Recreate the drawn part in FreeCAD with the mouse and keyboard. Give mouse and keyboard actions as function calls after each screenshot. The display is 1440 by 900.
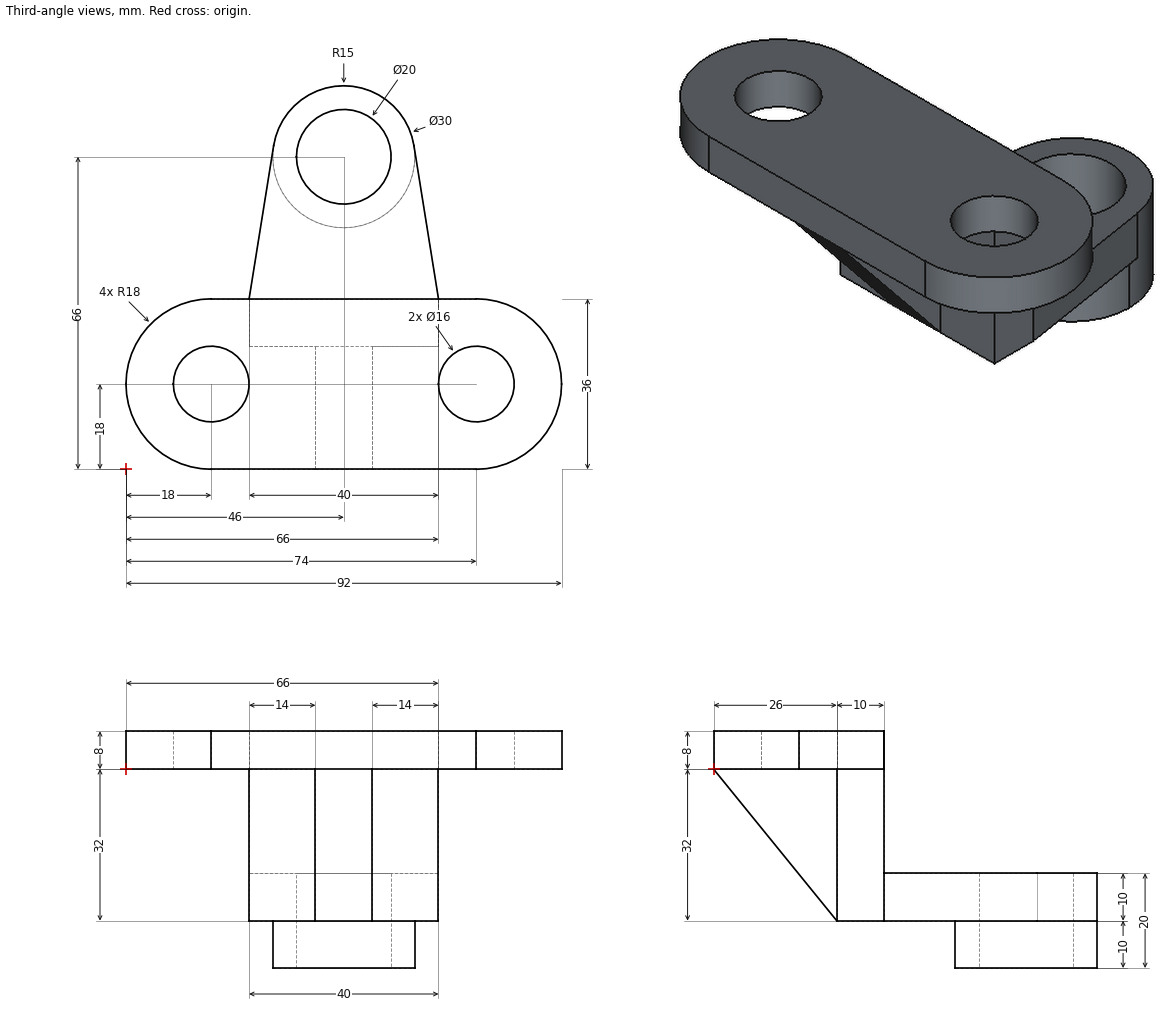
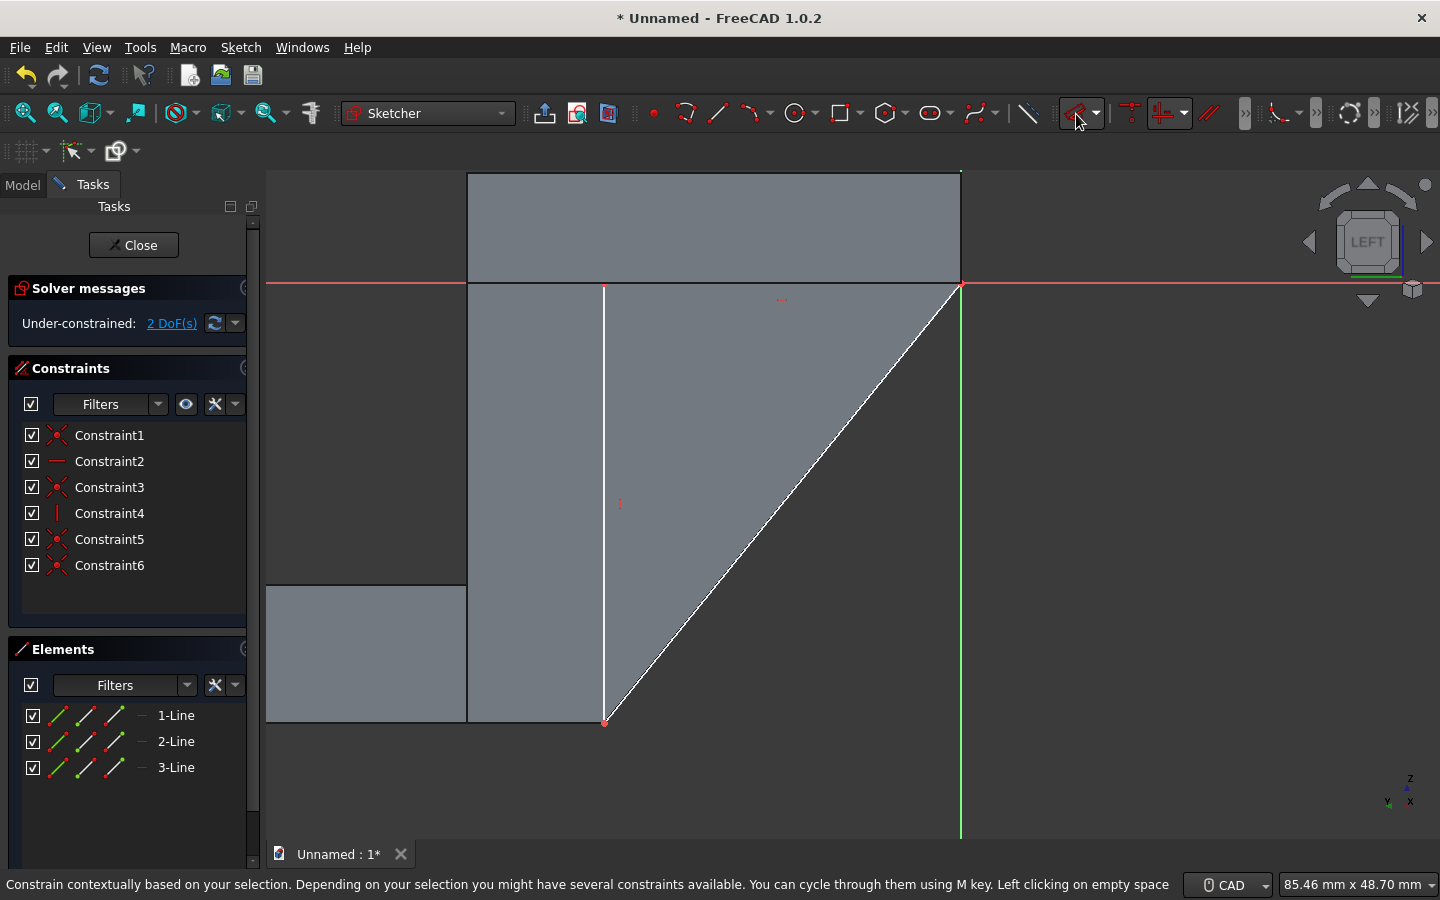
click(854, 283)
click(783, 249)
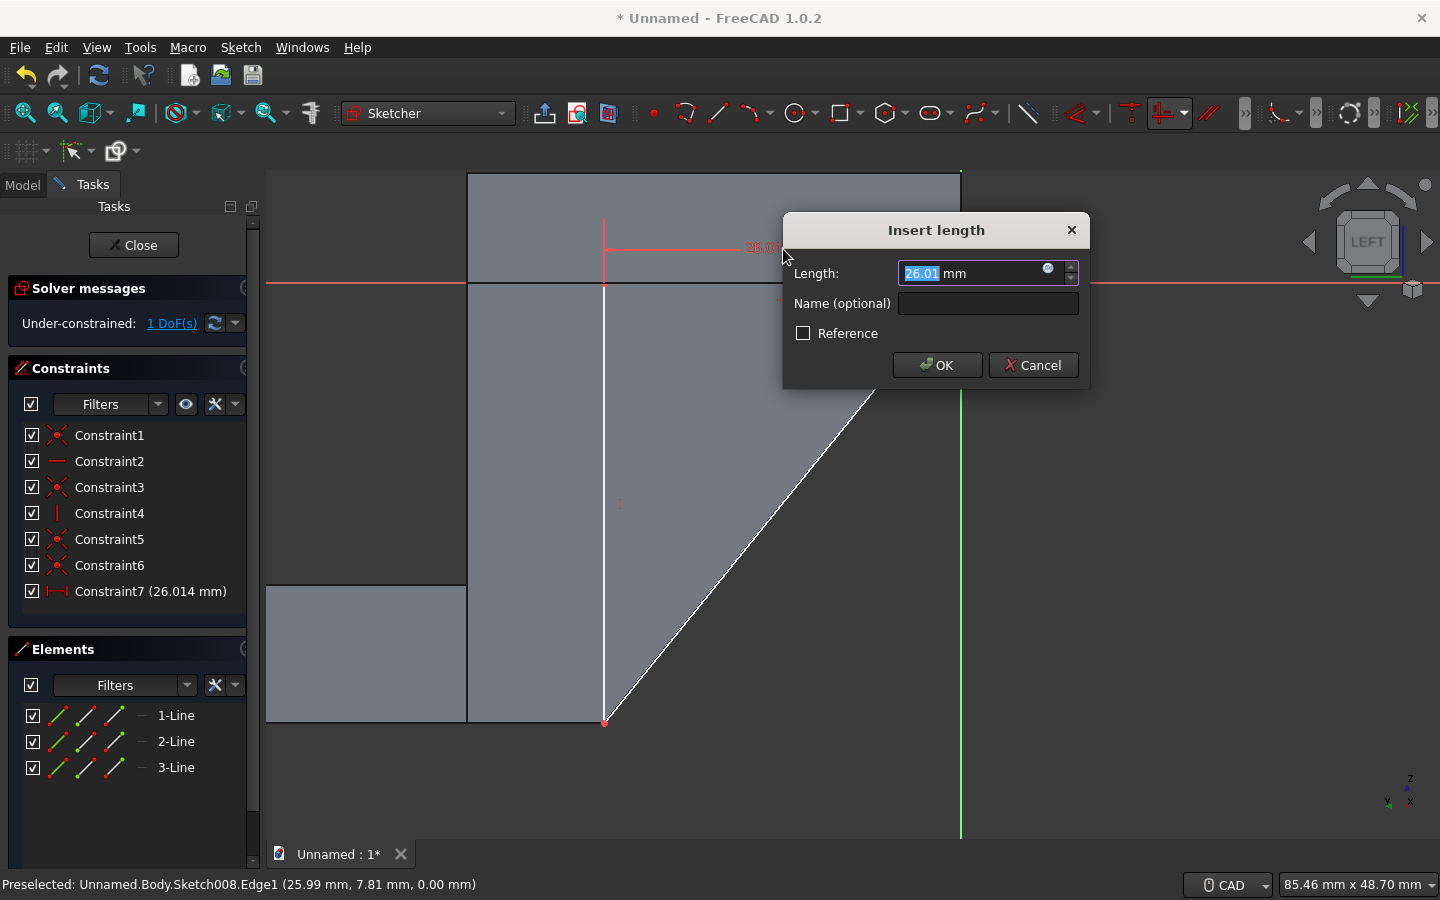
text(26)
key(Return)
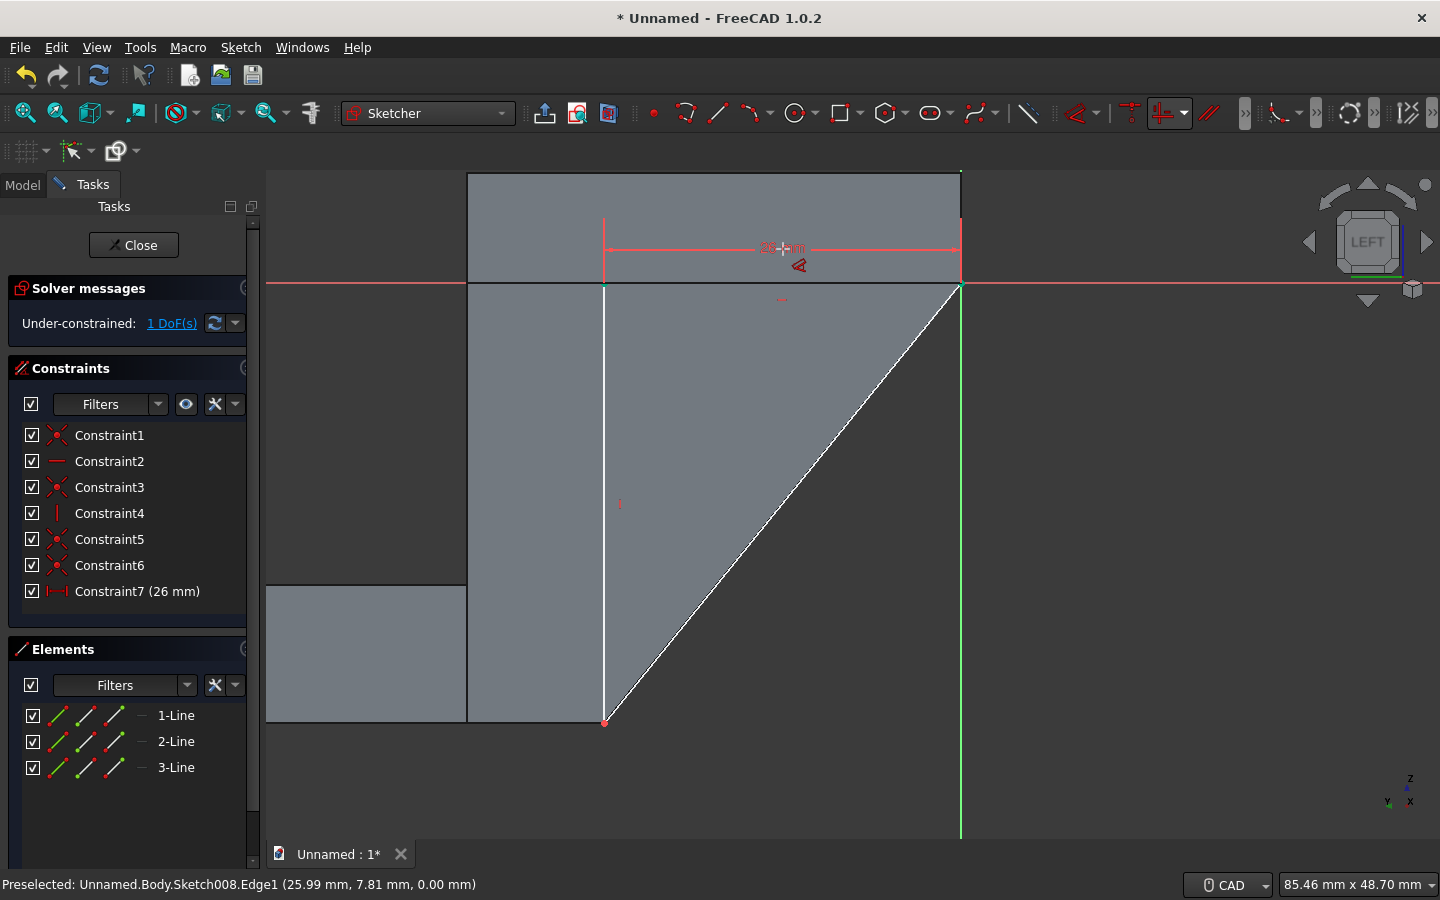
click(604, 415)
click(570, 504)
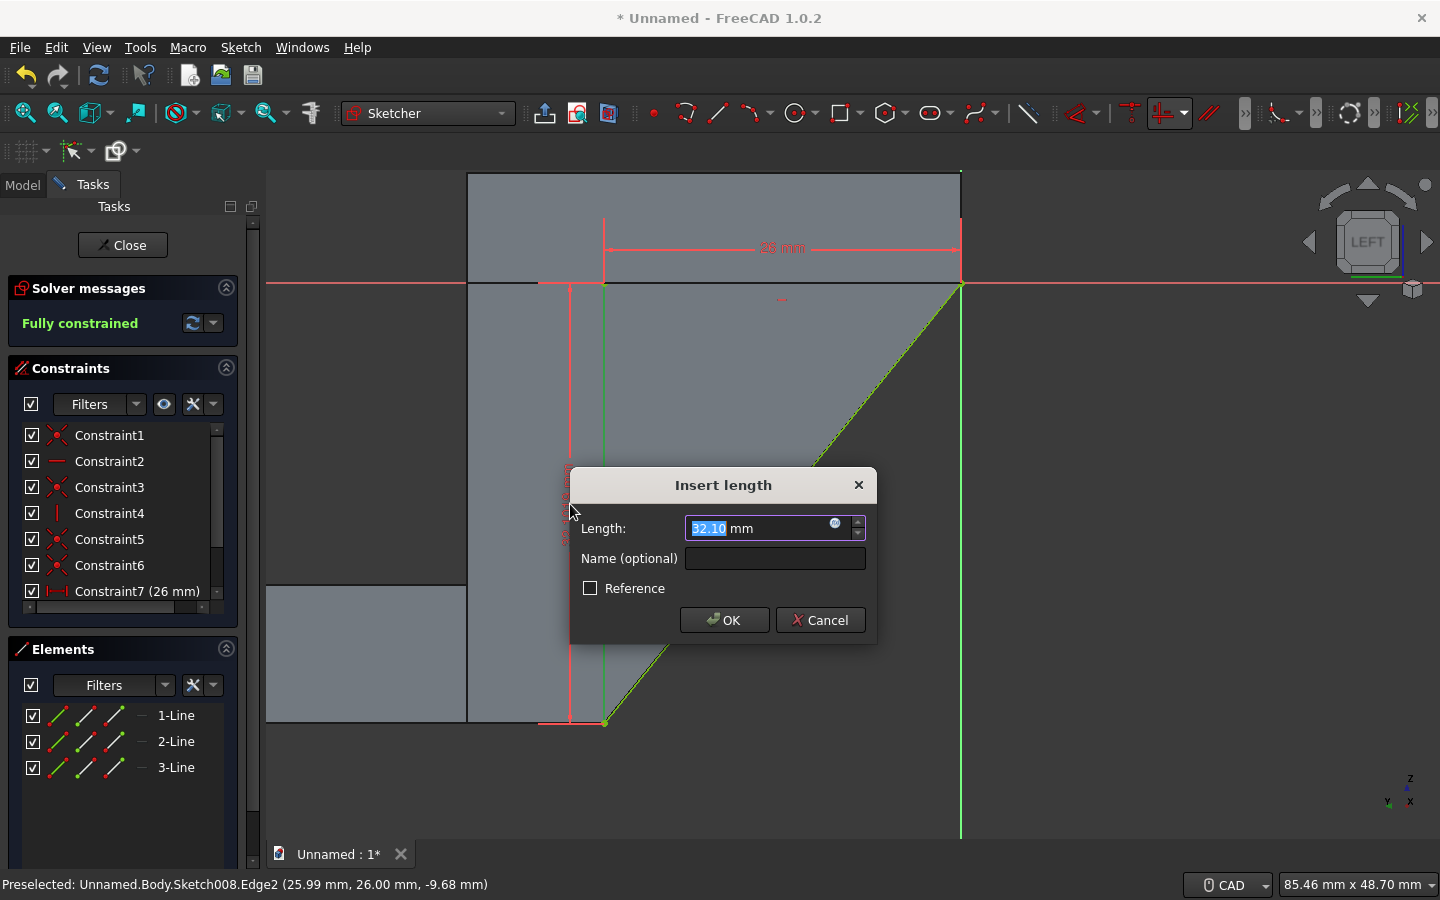
text(32)
key(Return)
key(Escape)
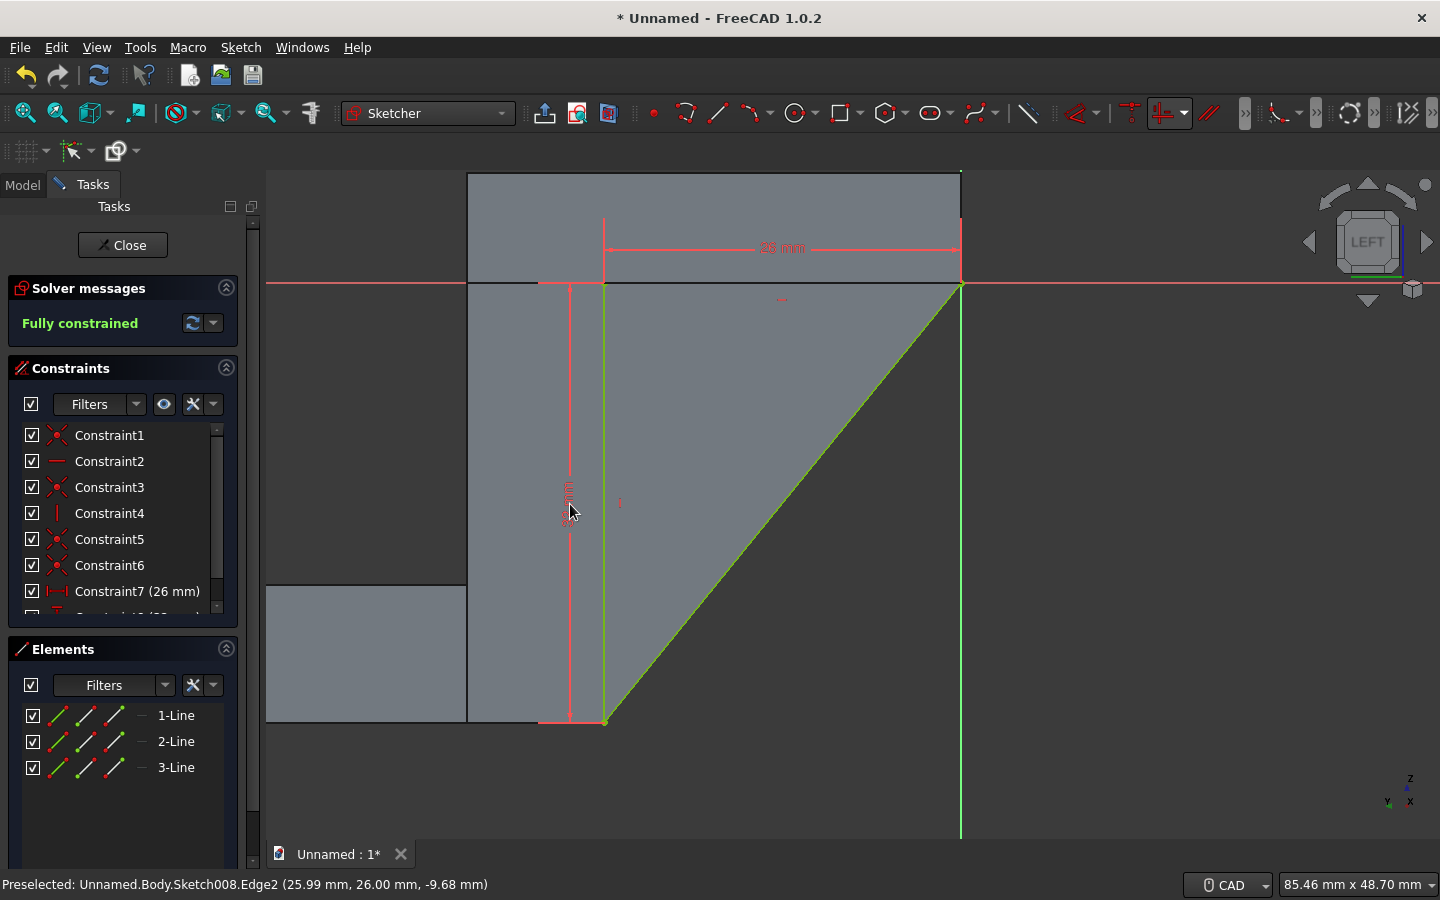
click(123, 245)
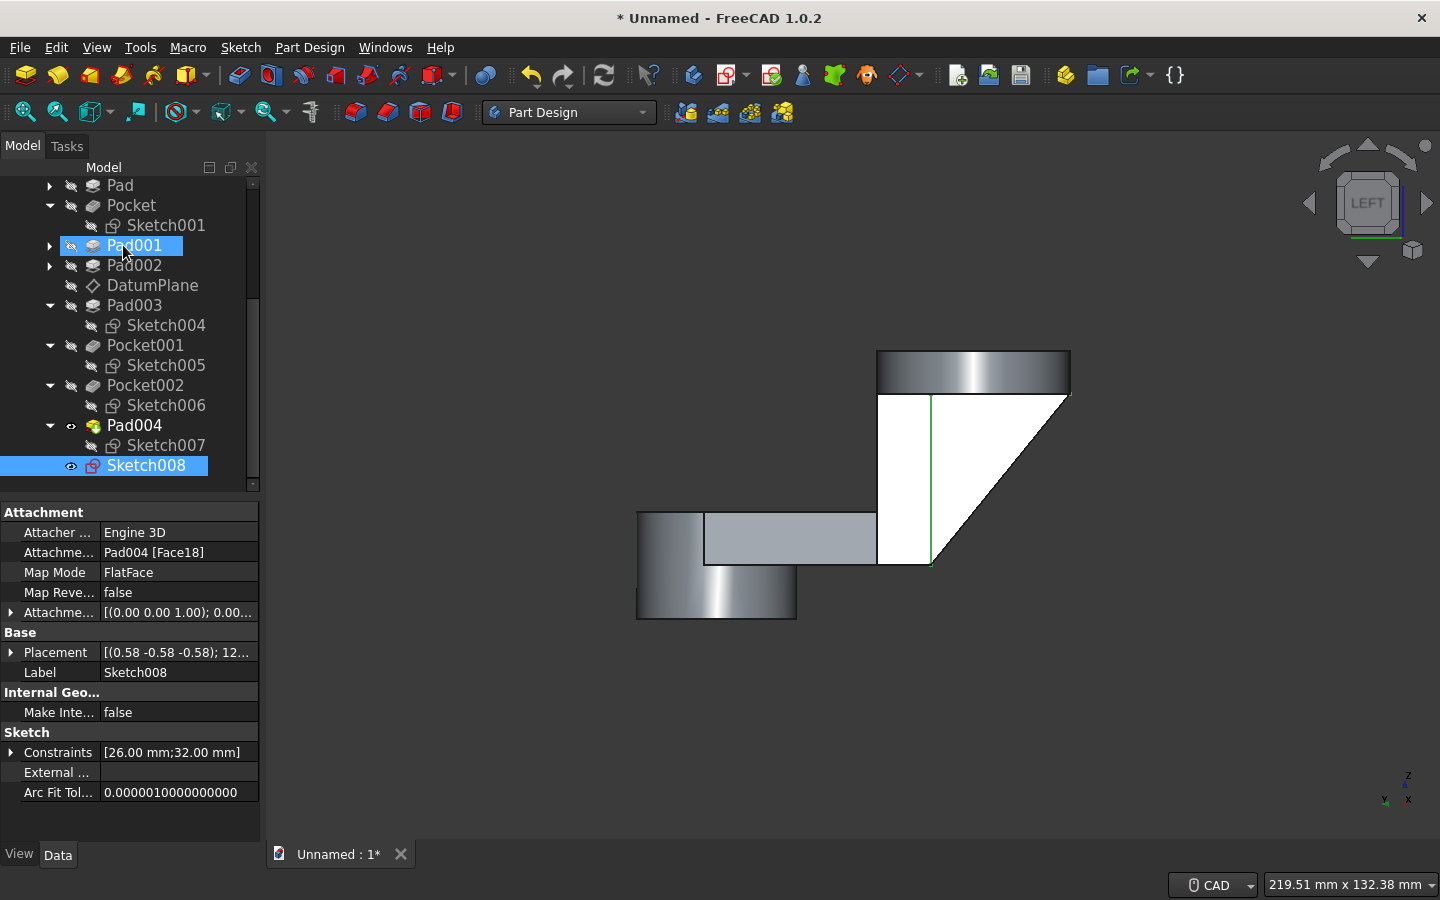
click(240, 76)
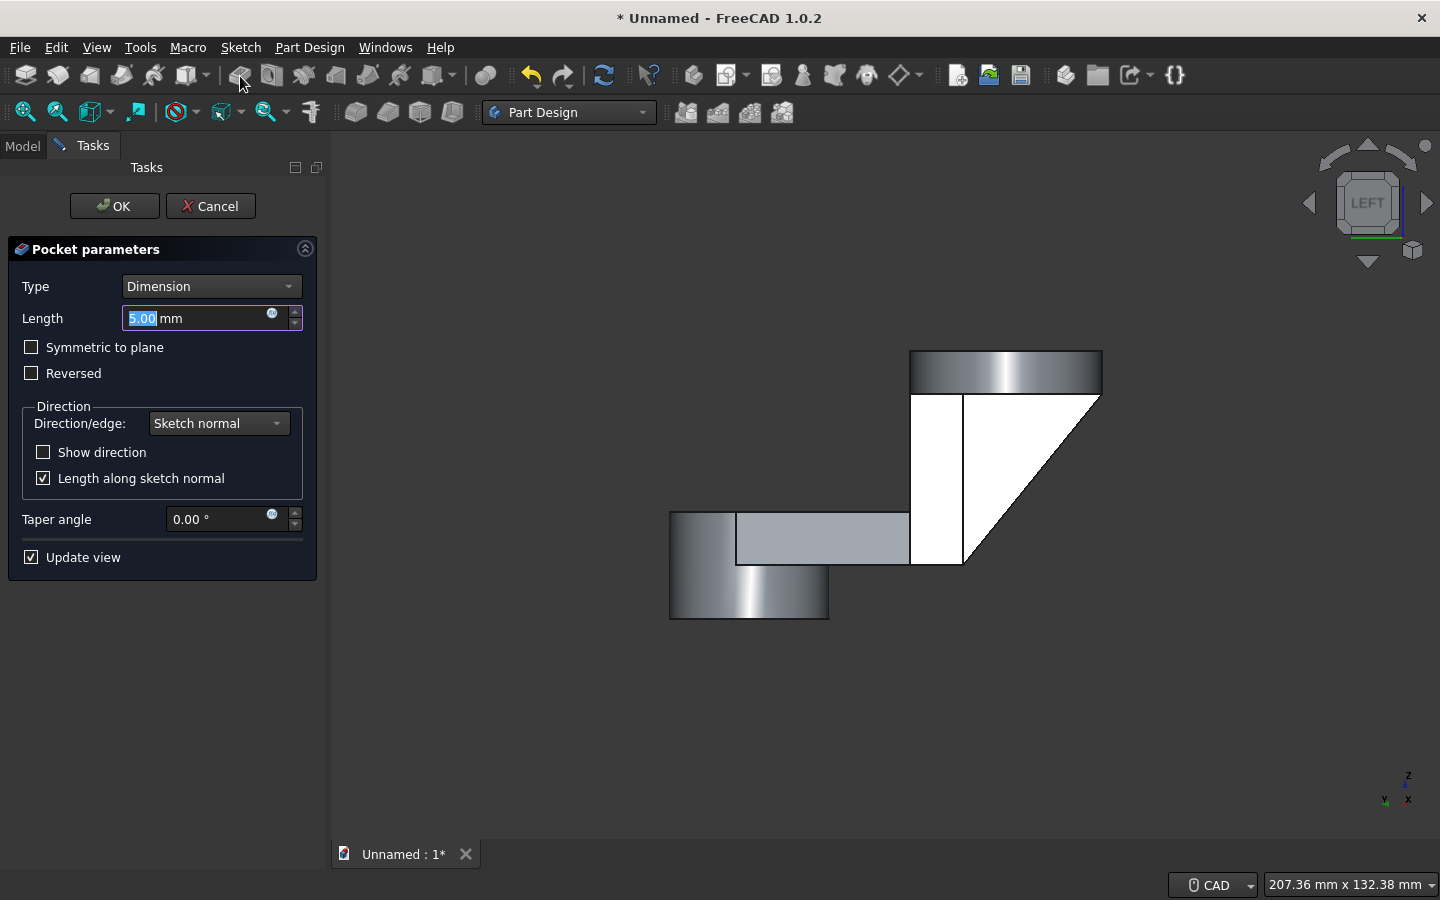
text(14)
key(Tab)